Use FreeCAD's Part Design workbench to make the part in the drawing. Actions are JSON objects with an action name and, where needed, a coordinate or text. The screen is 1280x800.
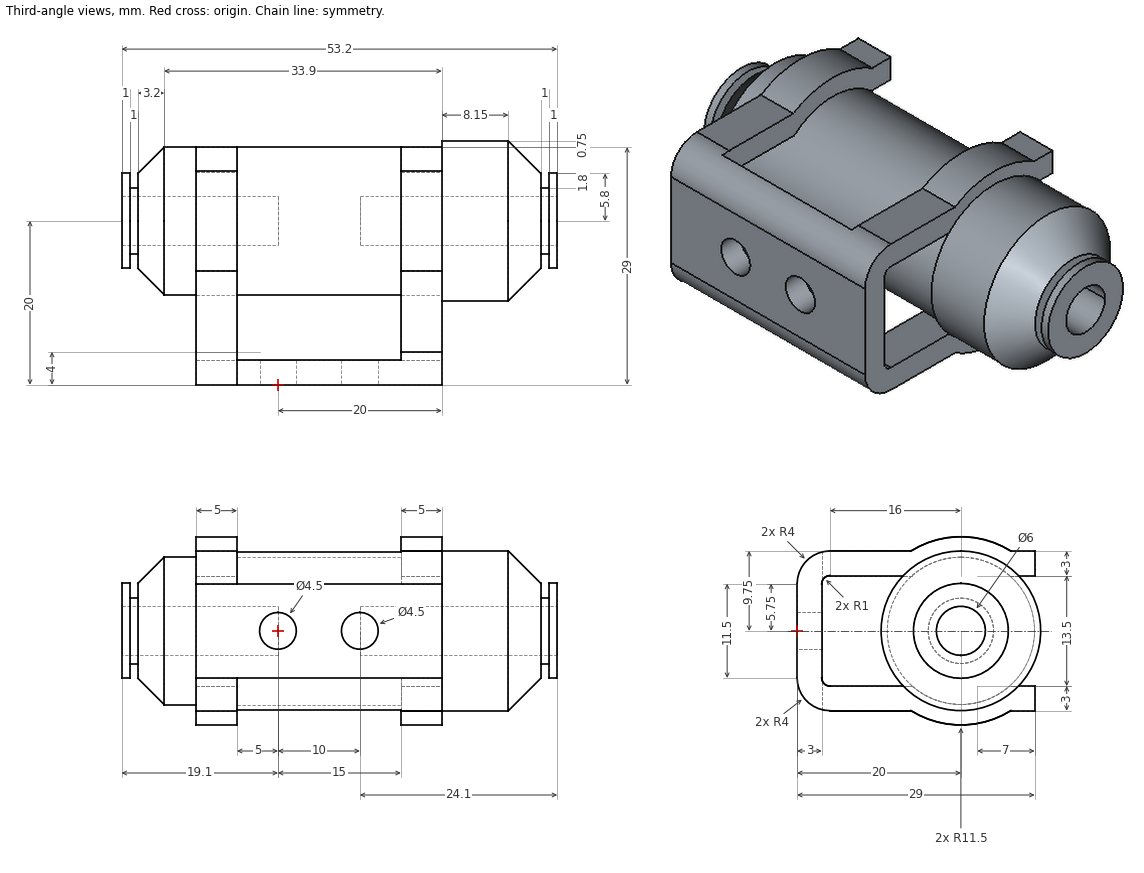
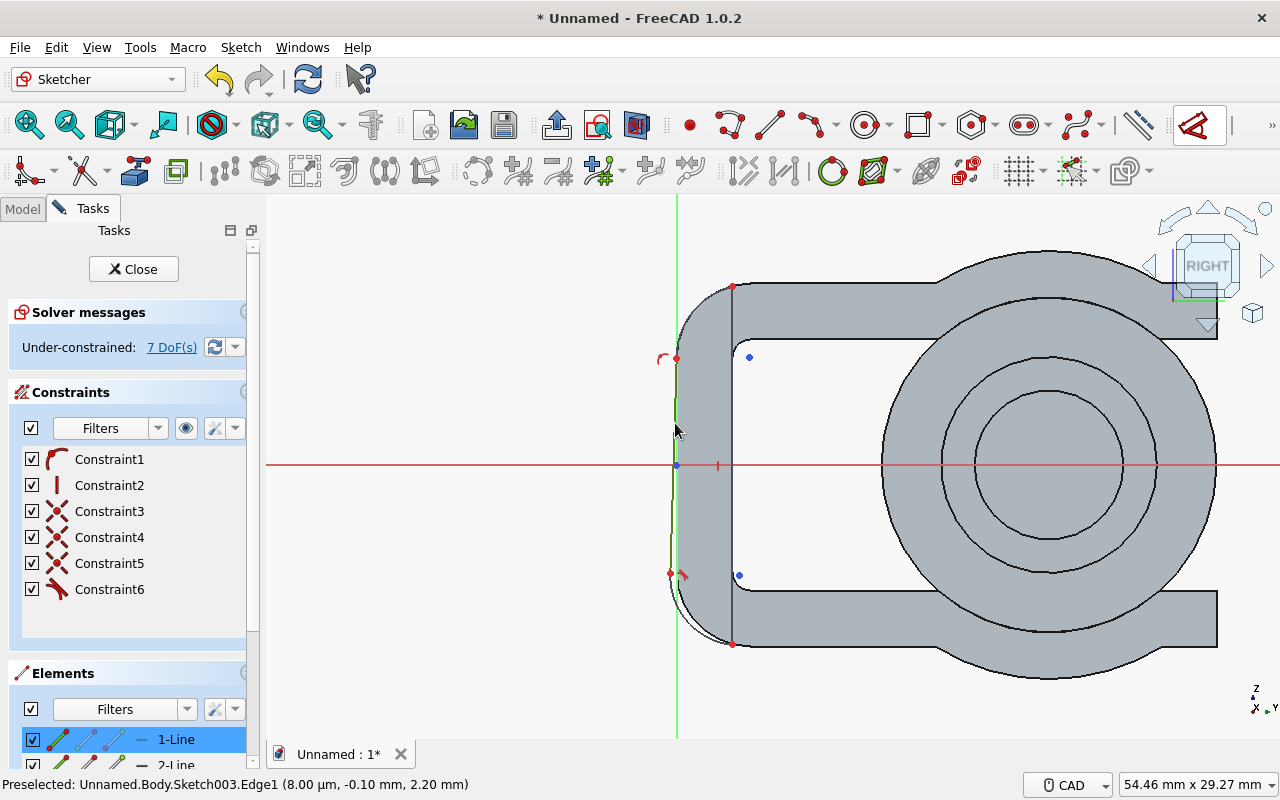
{"action": "left_click", "coordinate": [706, 300]}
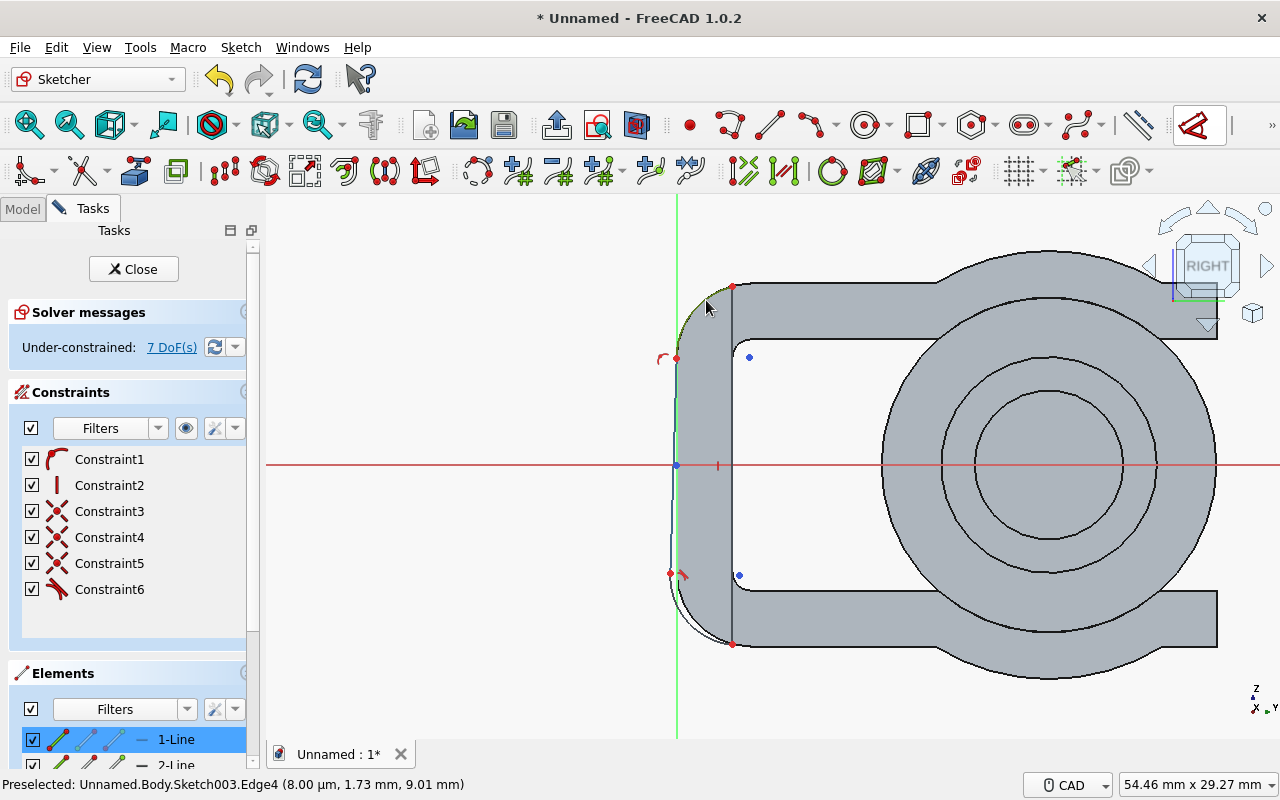
{"action": "key", "text": "t"}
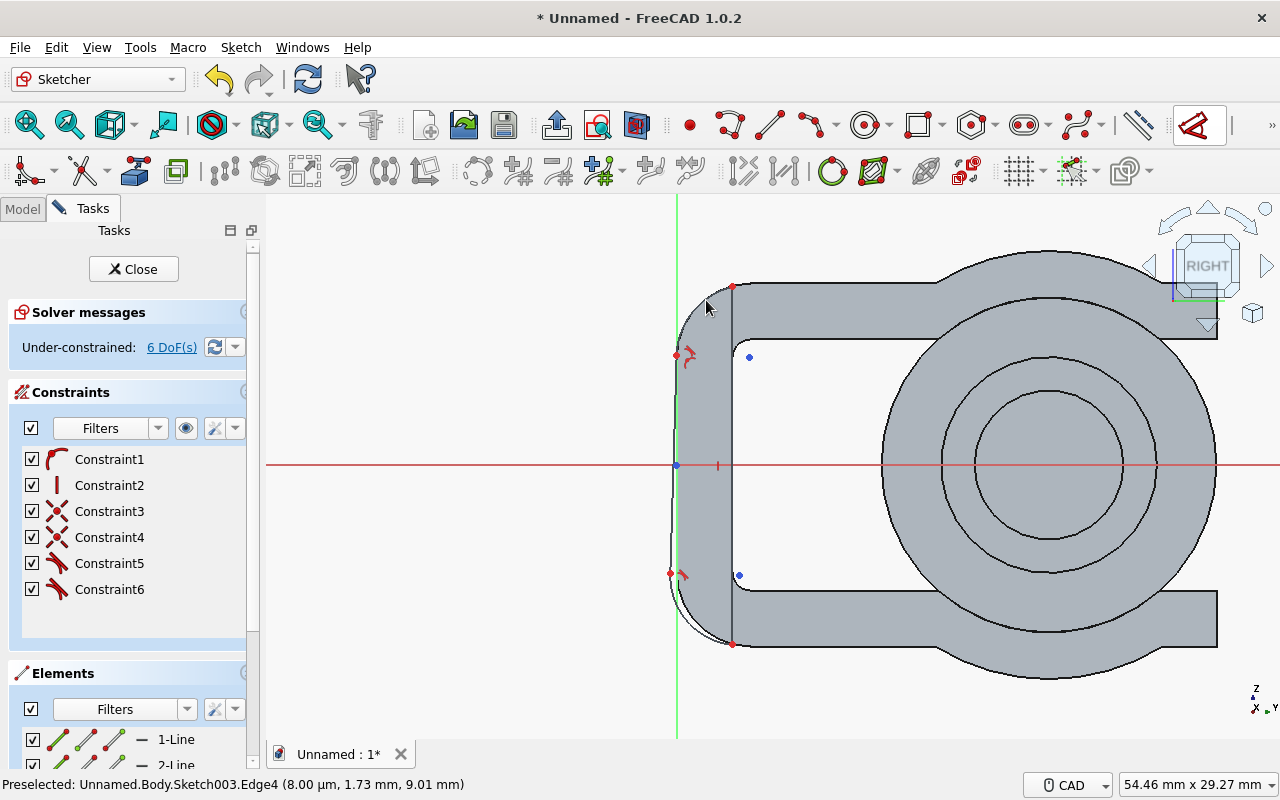
{"action": "left_click", "coordinate": [675, 421]}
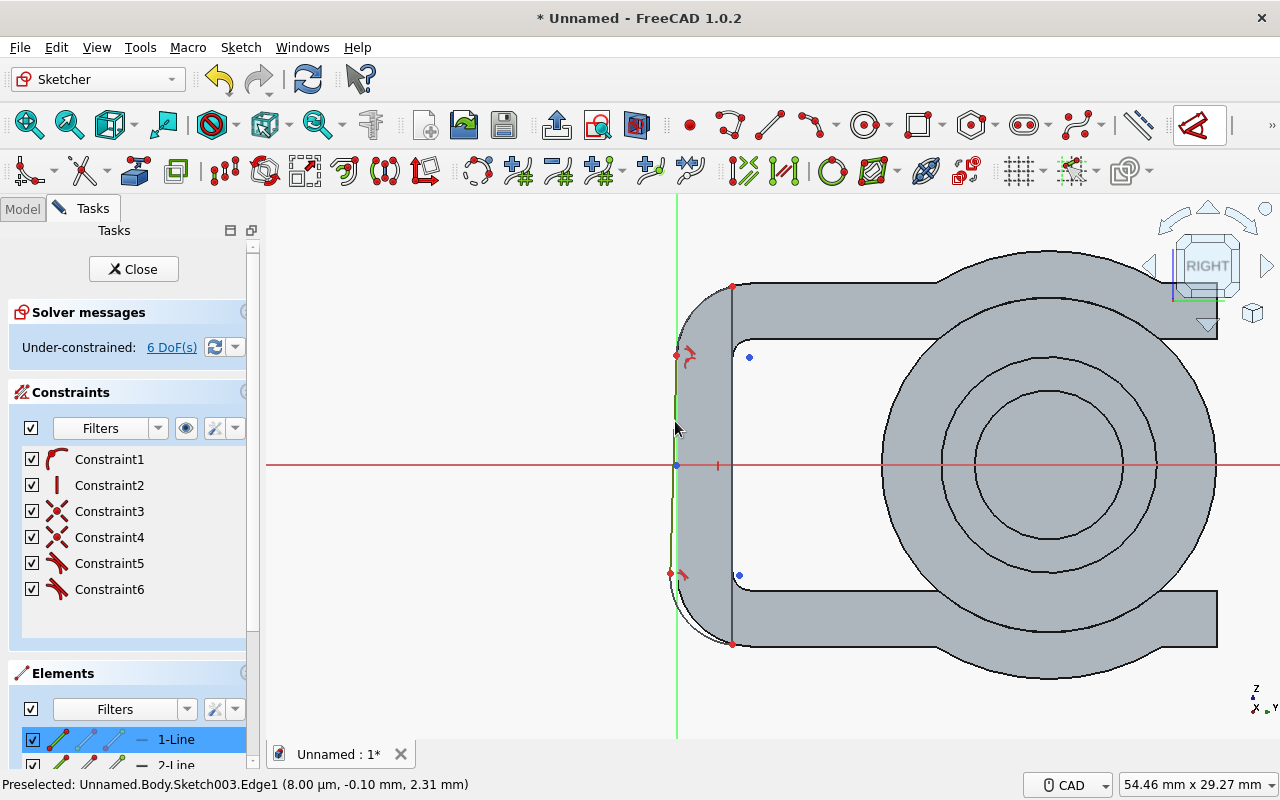
{"action": "key", "text": "v"}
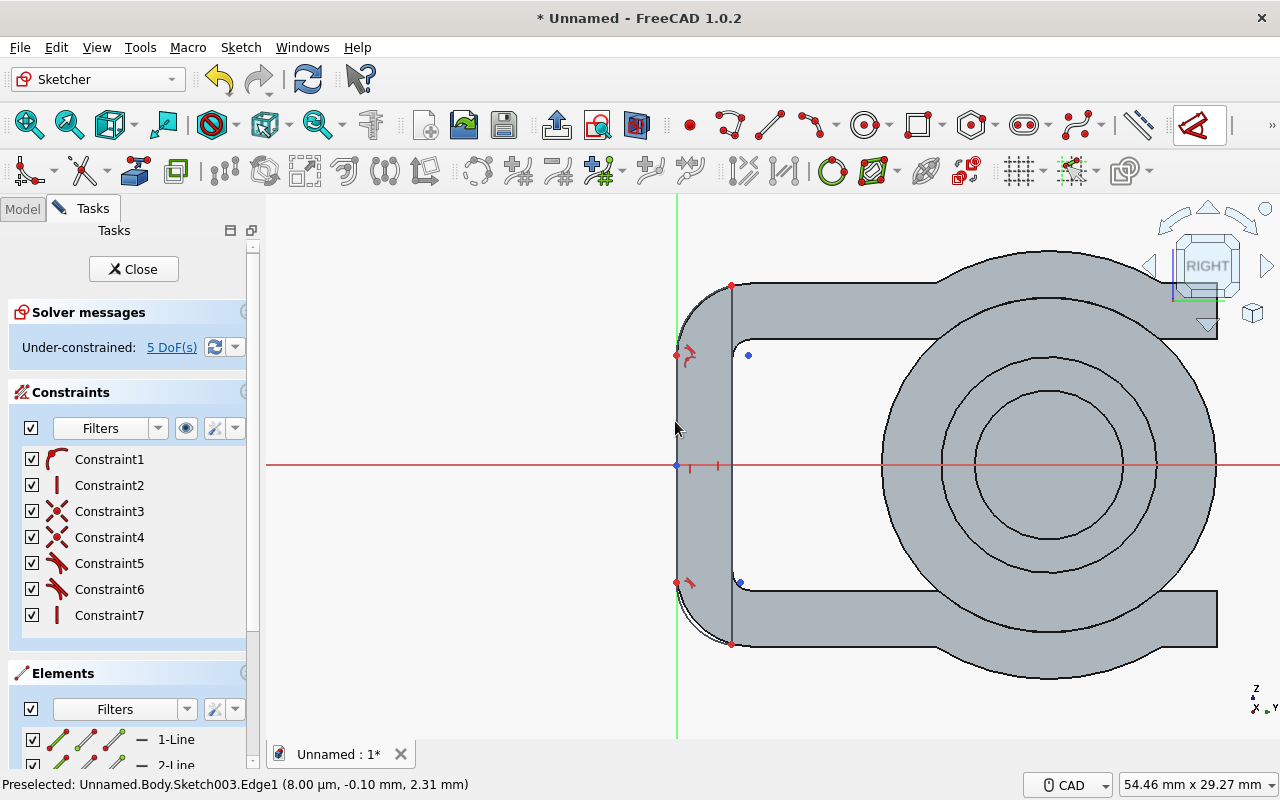
{"action": "left_click", "coordinate": [706, 636]}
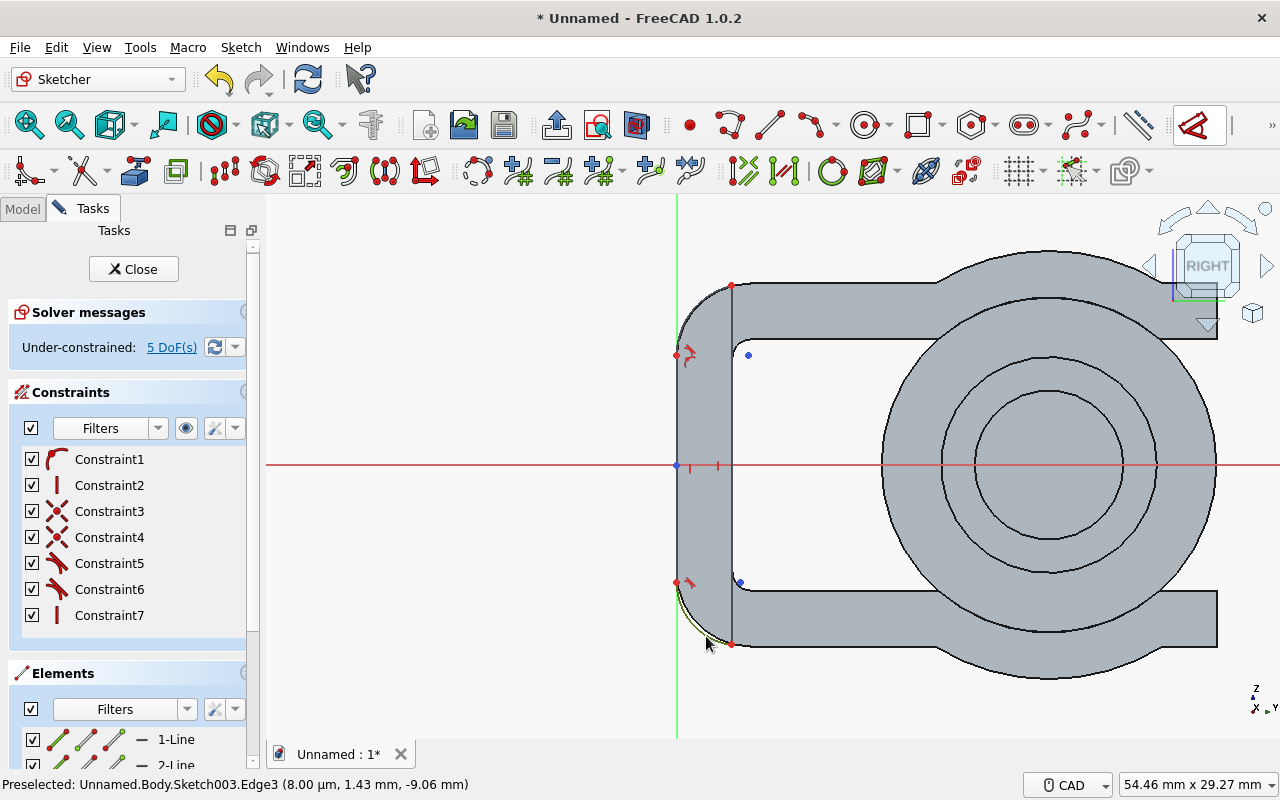
{"action": "left_click", "coordinate": [706, 298]}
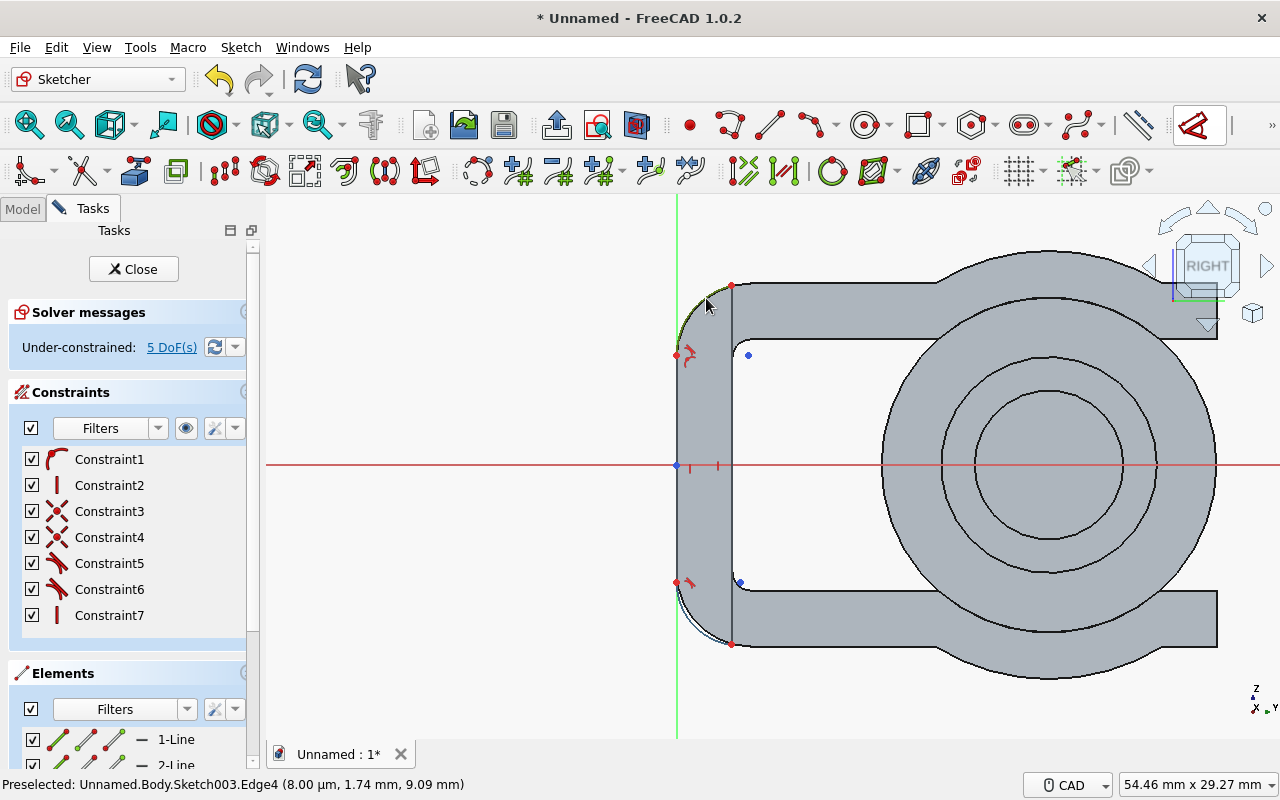
{"action": "key", "text": "e"}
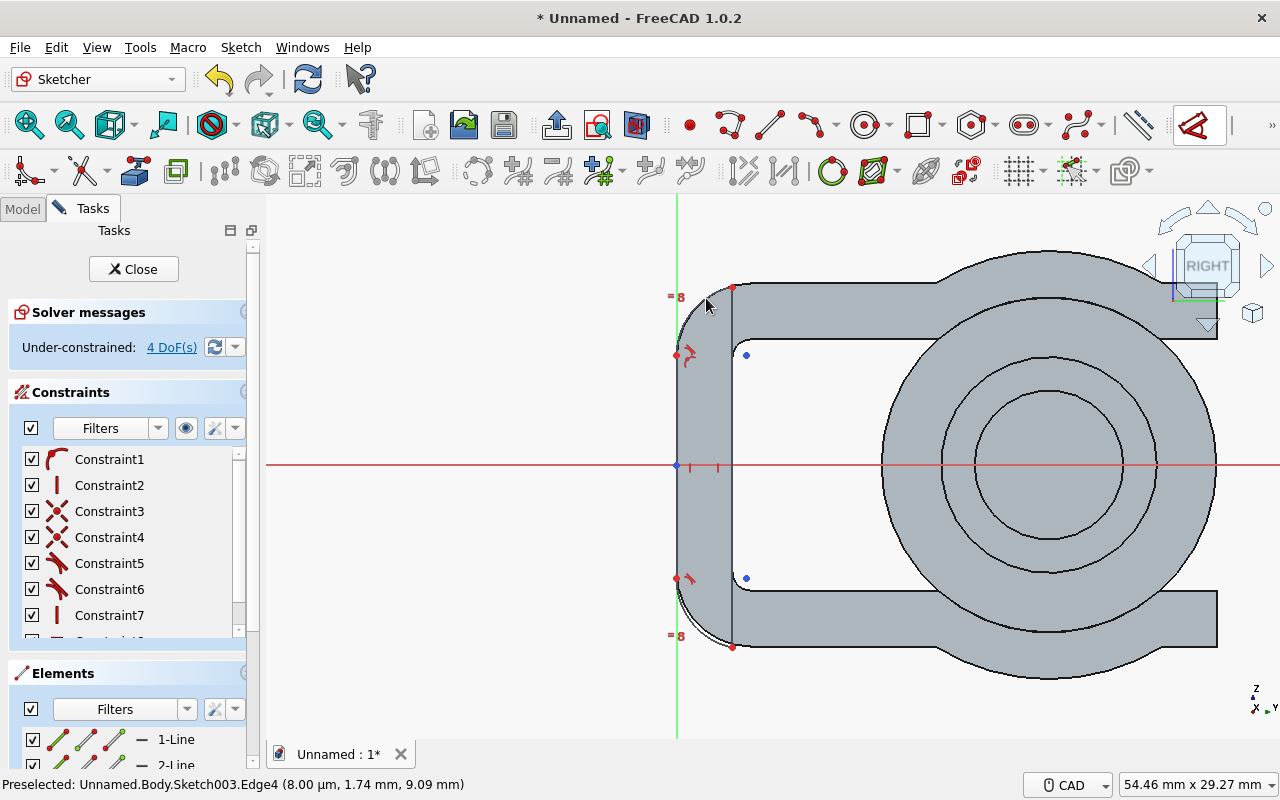
{"action": "left_click", "coordinate": [706, 636]}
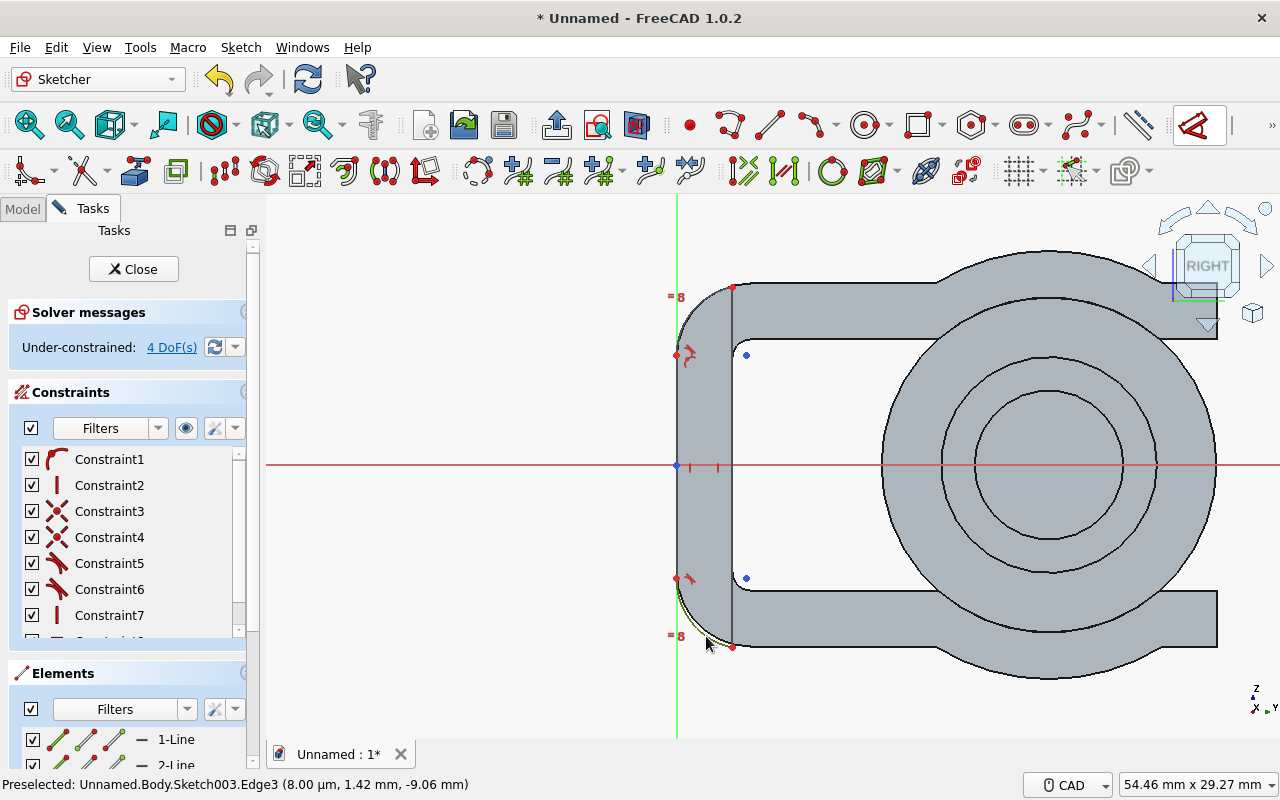
{"action": "key", "text": "k r"}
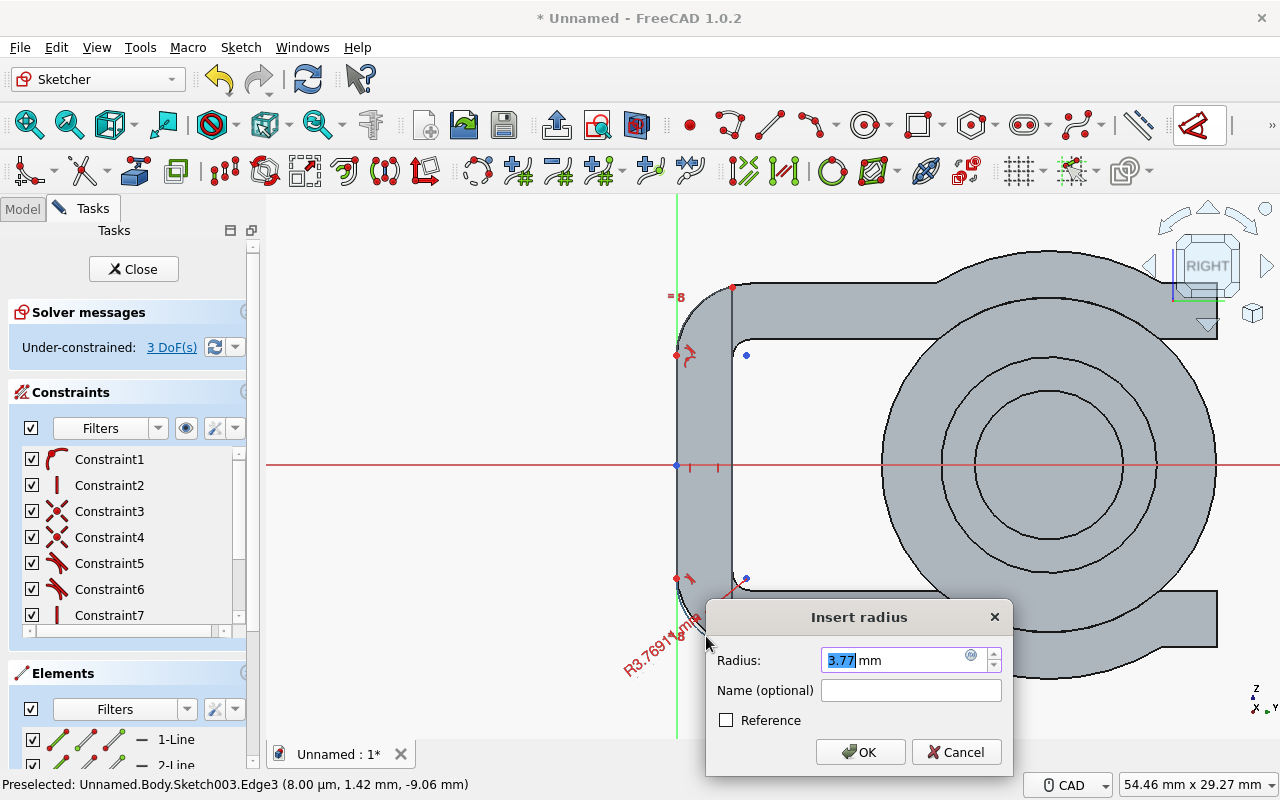
{"action": "type", "text": "4"}
{"action": "key", "text": "Return"}